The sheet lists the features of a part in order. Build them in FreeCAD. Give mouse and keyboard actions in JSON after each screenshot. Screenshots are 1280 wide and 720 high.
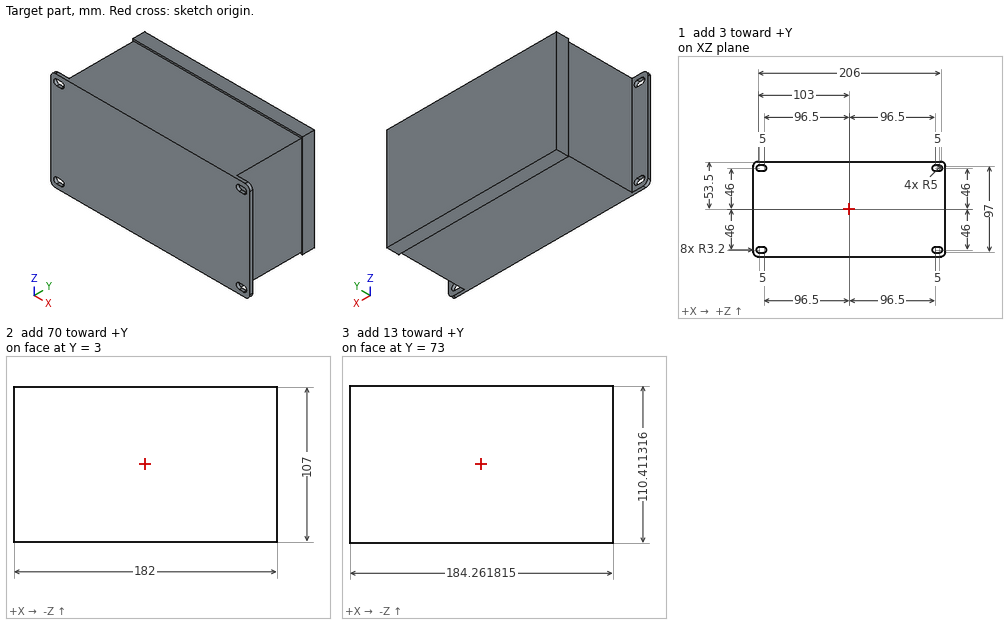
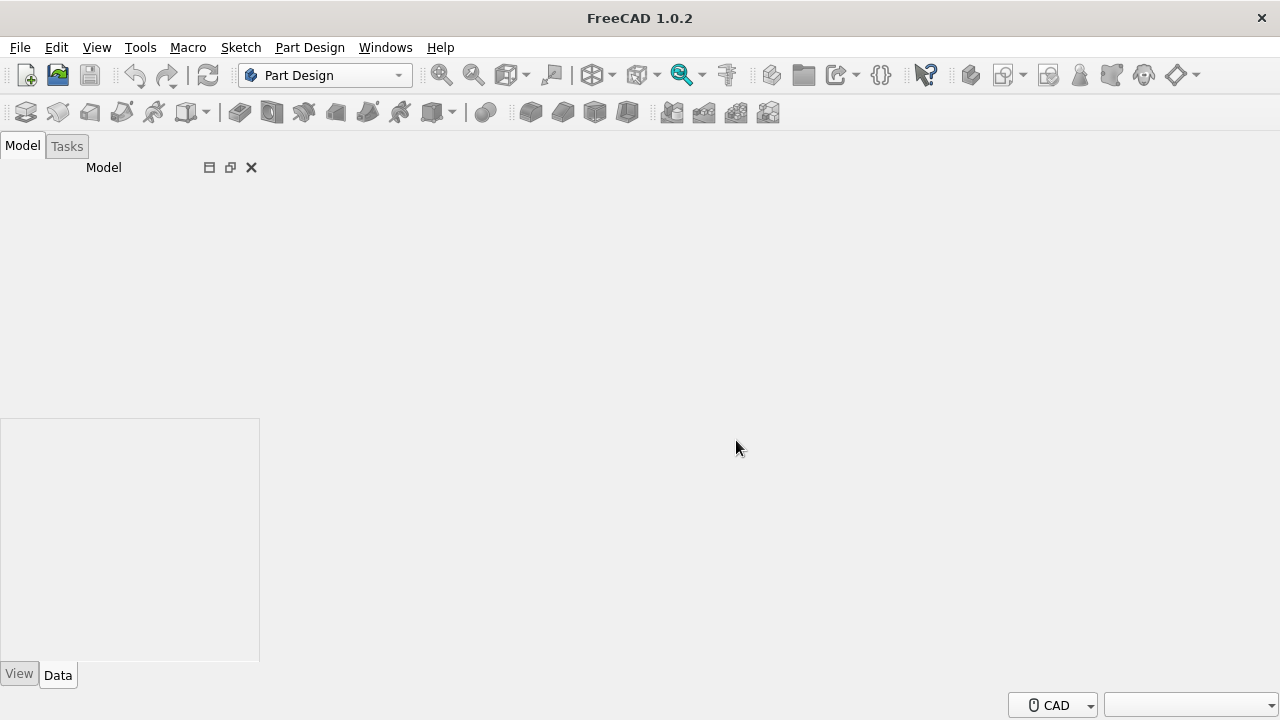
{"action": "left_click", "coordinate": [26, 76]}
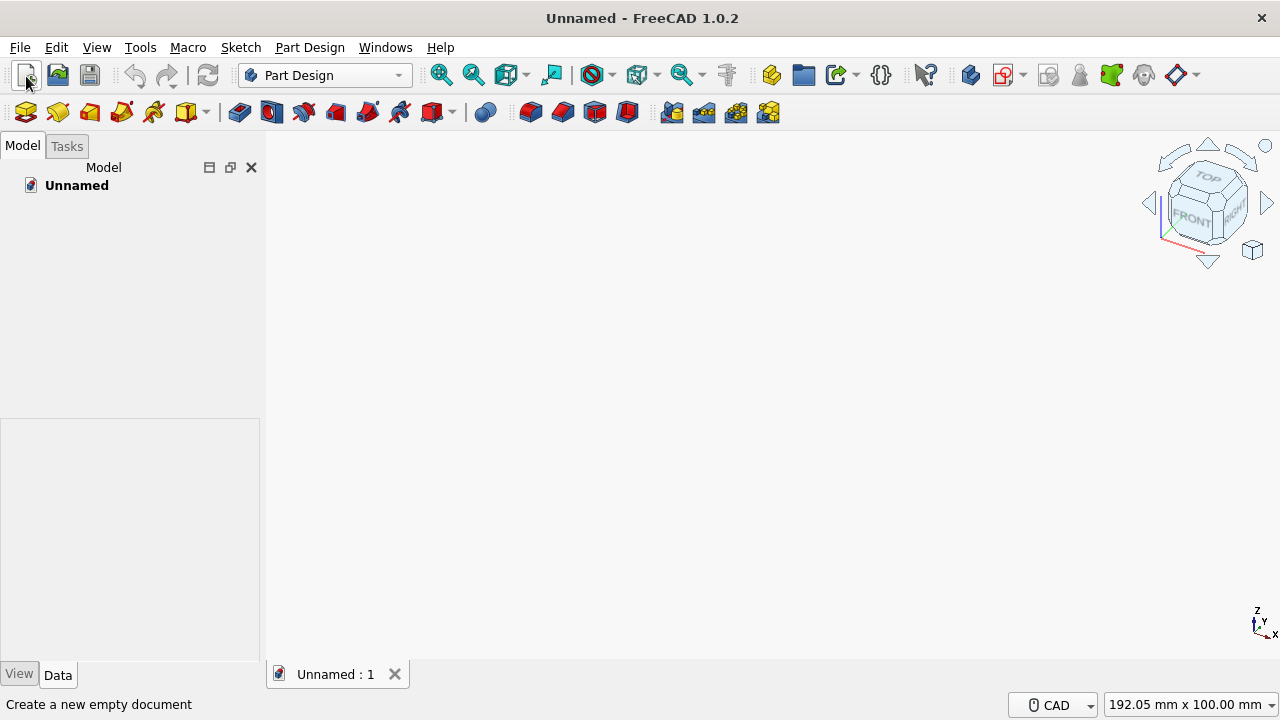
{"action": "left_click", "coordinate": [1004, 76]}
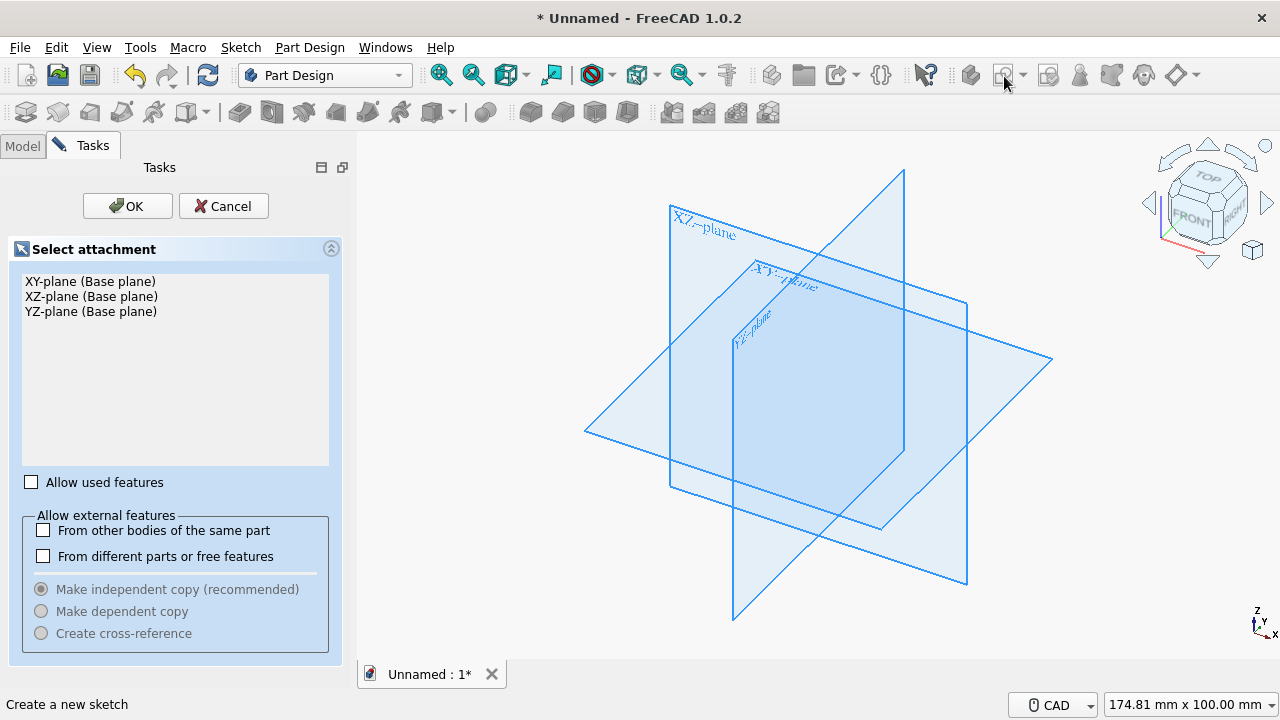
{"action": "left_click", "coordinate": [82, 296]}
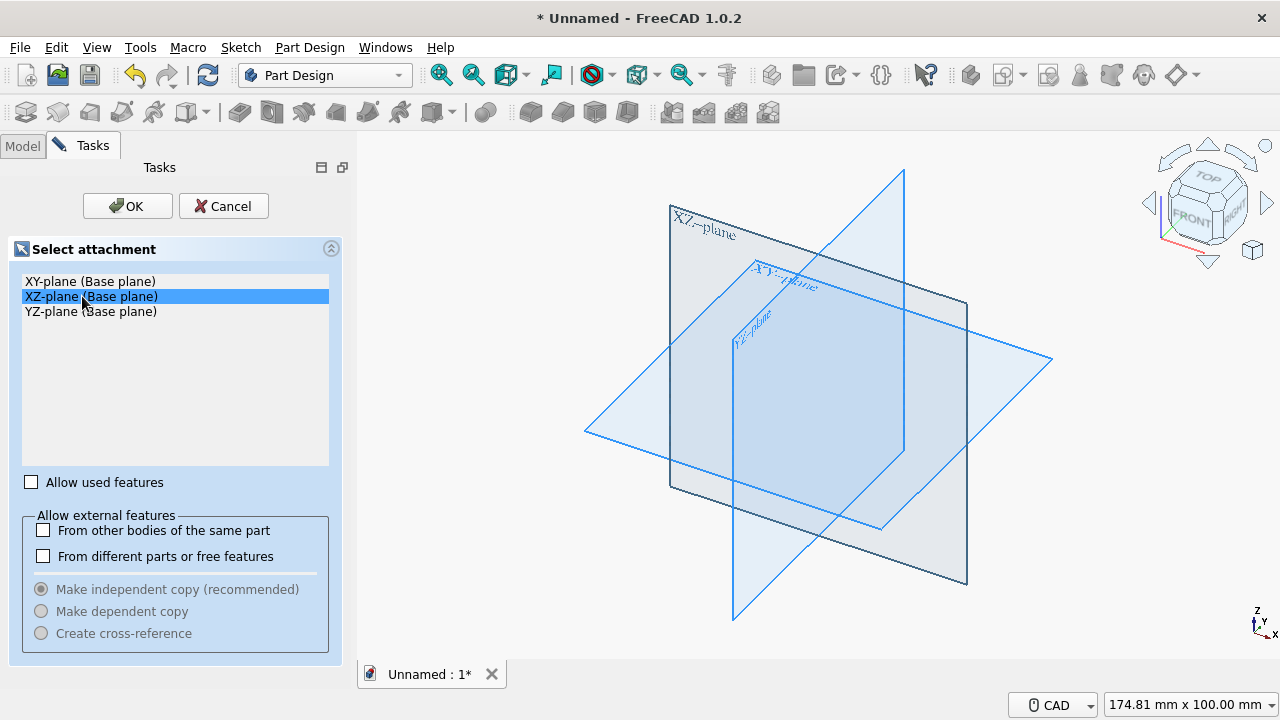
{"action": "left_click", "coordinate": [128, 206]}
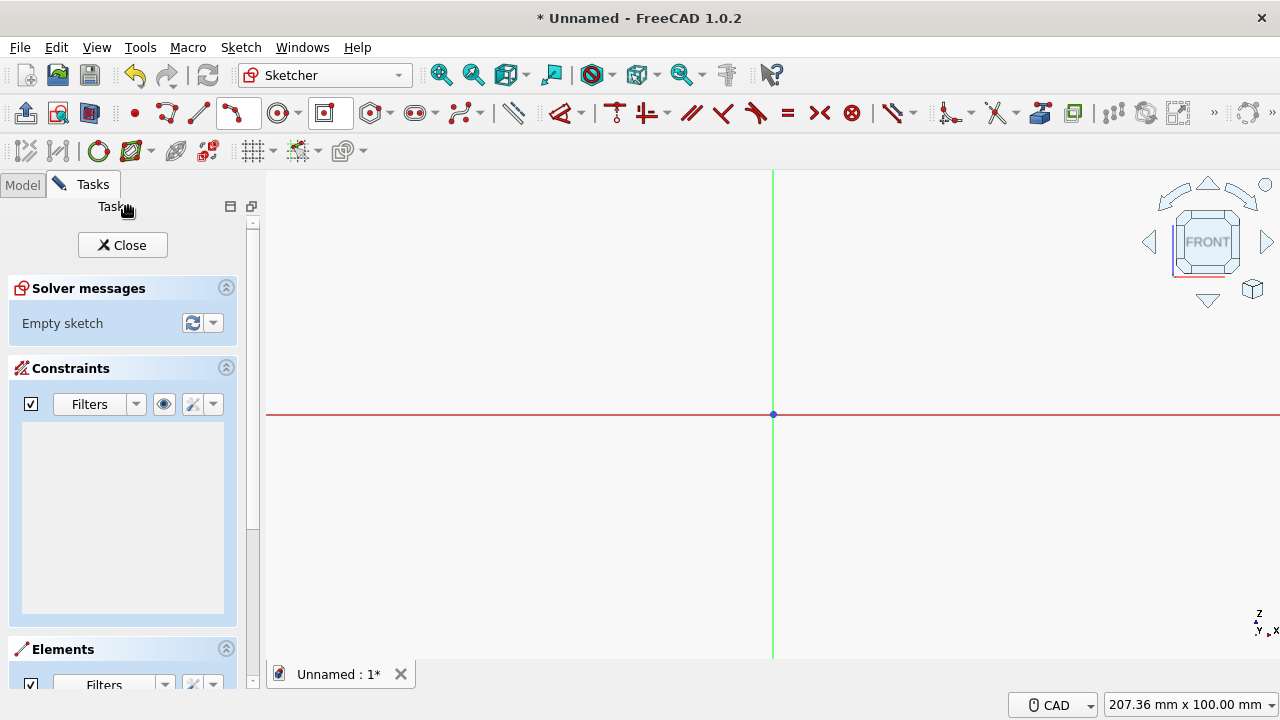
{"action": "scroll", "coordinate": [621, 414], "scroll_direction": "down", "scroll_amount": 3}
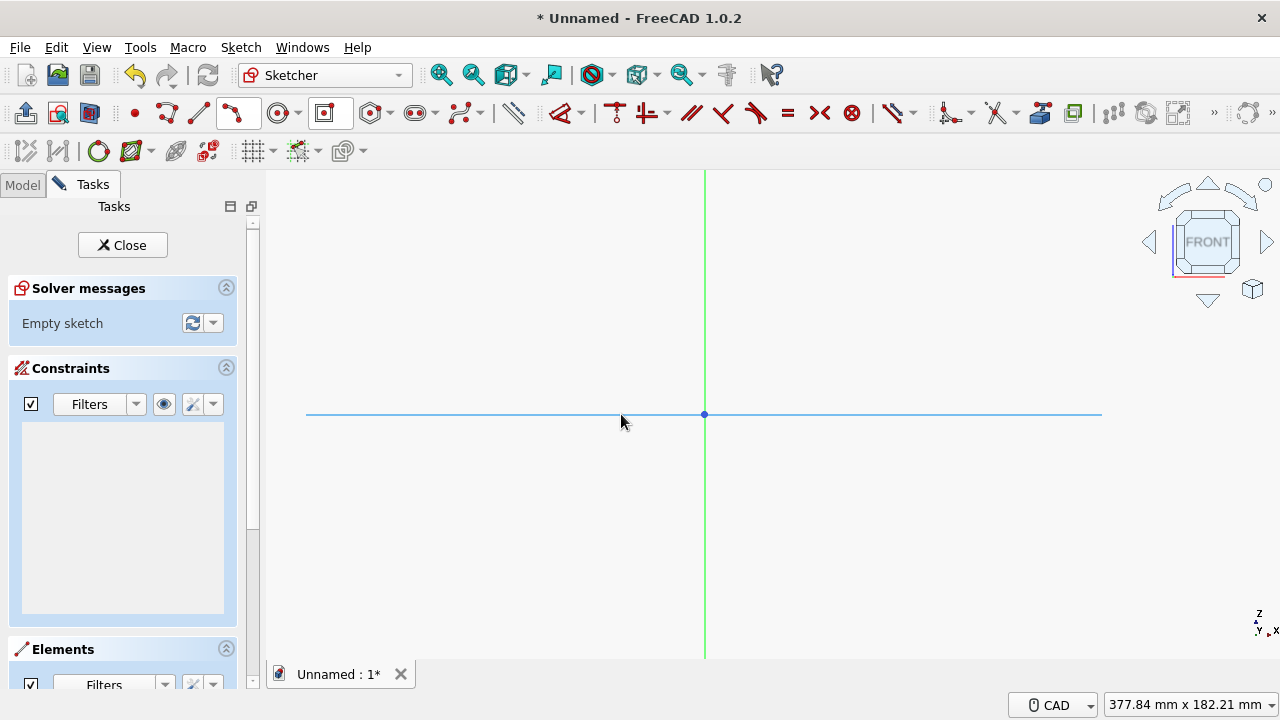
{"action": "left_click", "coordinate": [200, 114]}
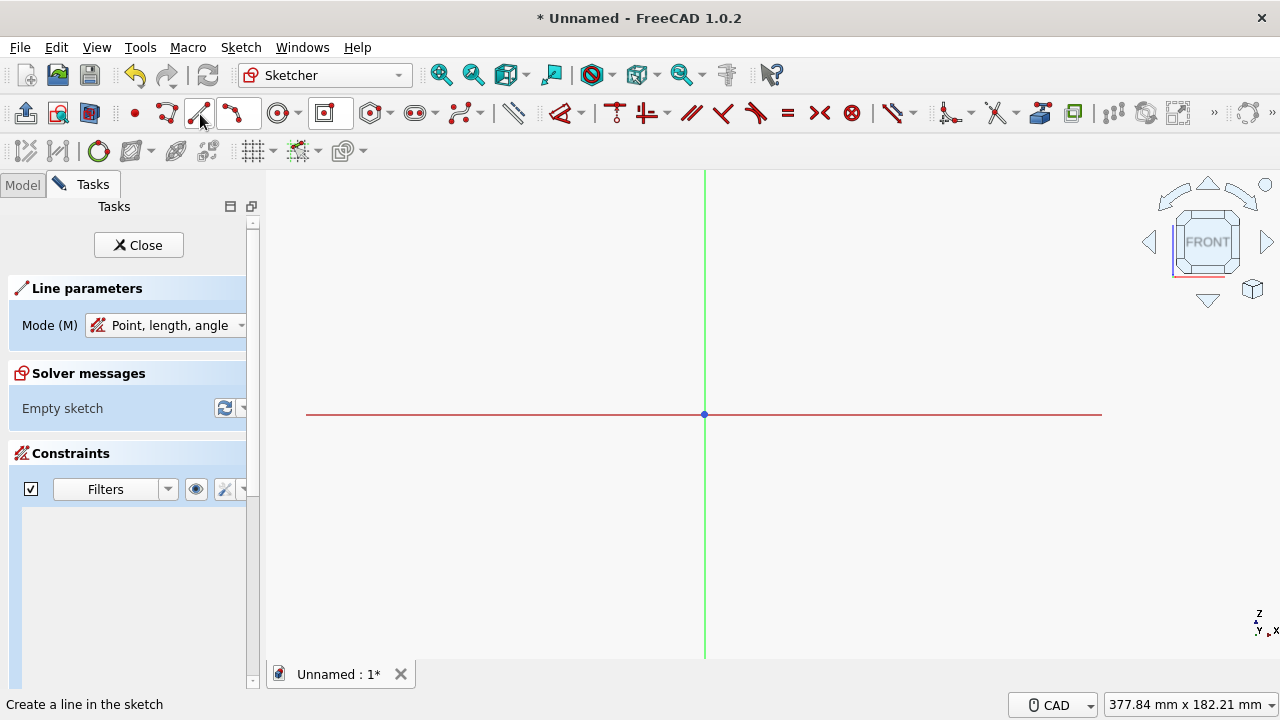
{"action": "left_click", "coordinate": [428, 271]}
{"action": "left_click", "coordinate": [981, 271]}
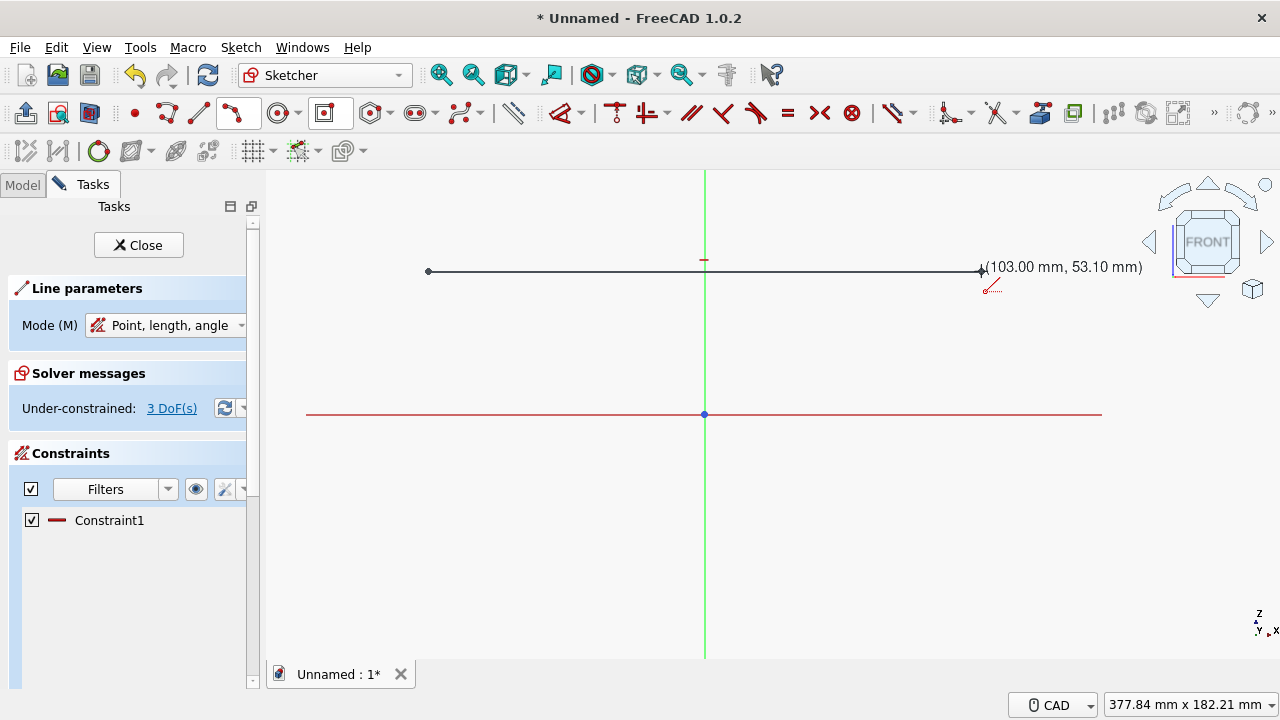
{"action": "left_click", "coordinate": [994, 284]}
{"action": "left_click", "coordinate": [994, 545]}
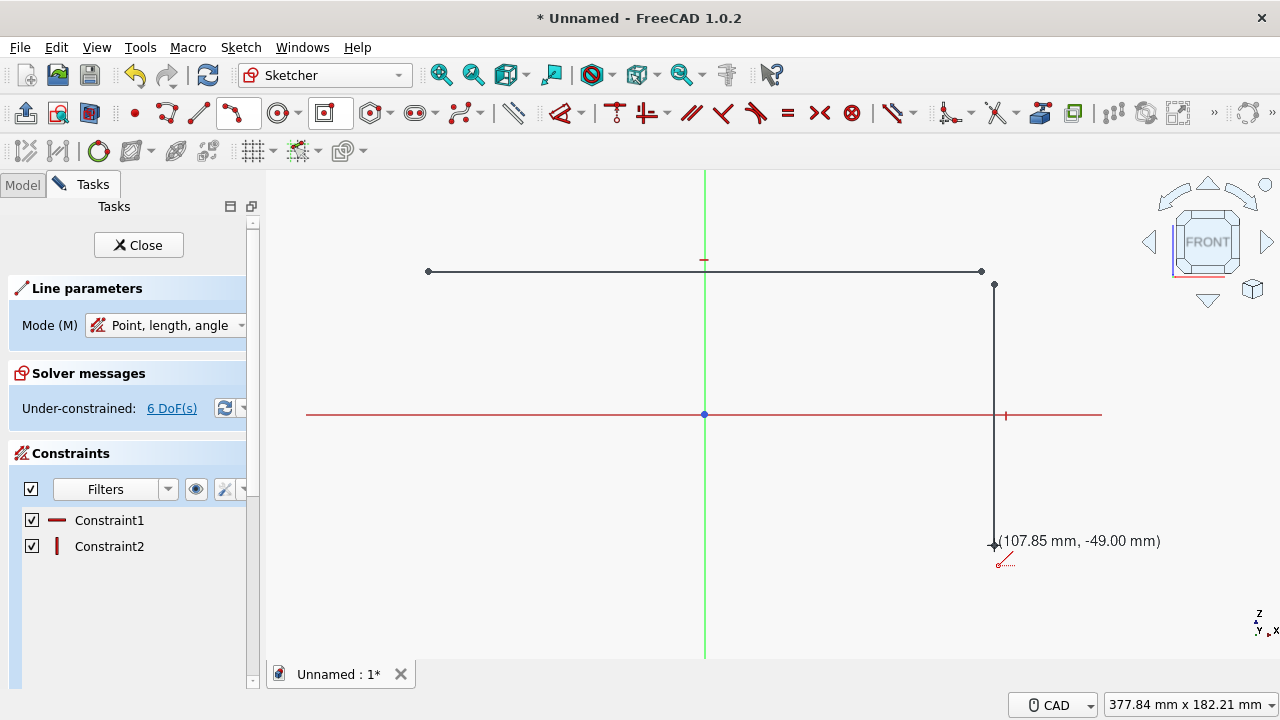
{"action": "left_click", "coordinate": [981, 558]}
{"action": "left_click", "coordinate": [428, 558]}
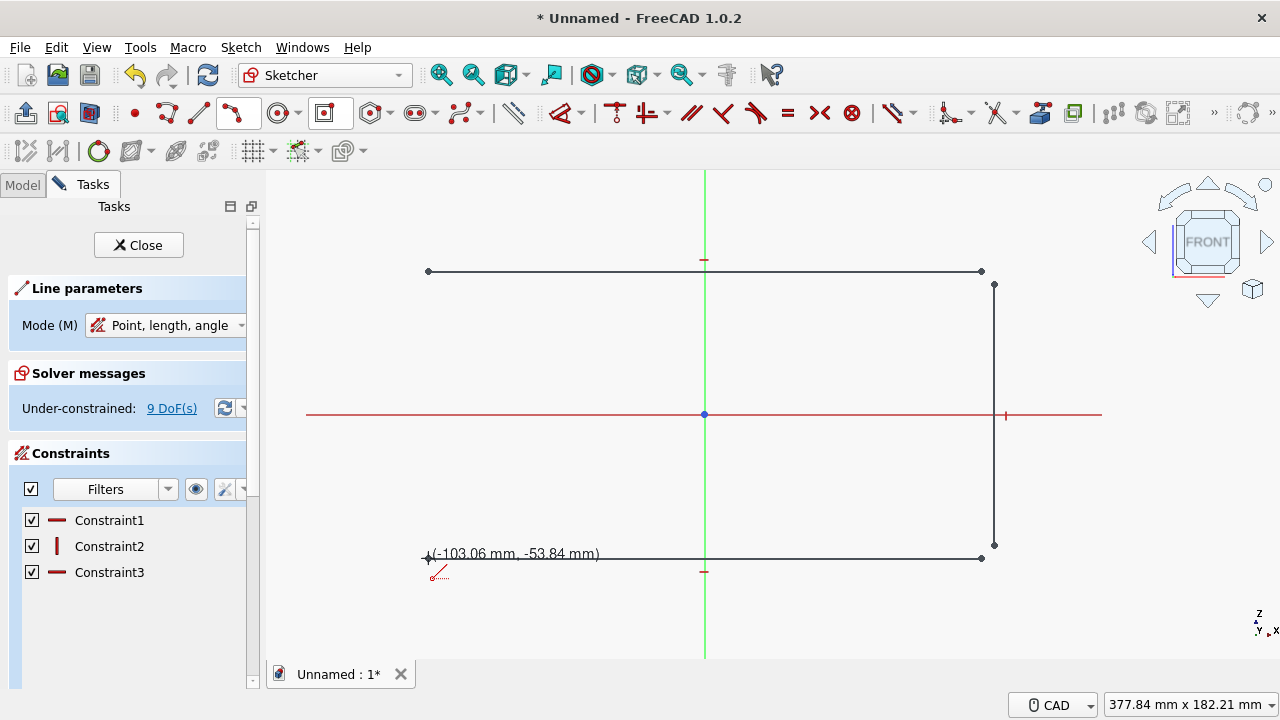
{"action": "left_click", "coordinate": [415, 545]}
{"action": "left_click", "coordinate": [415, 284]}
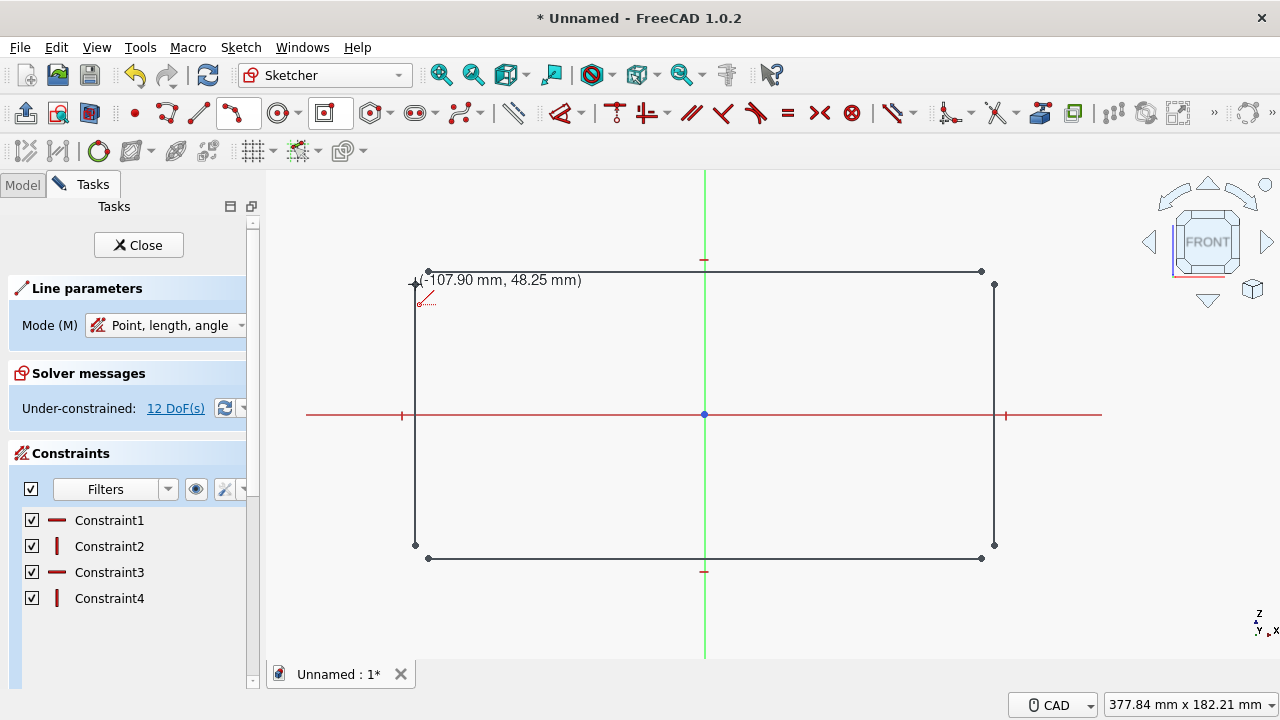
{"action": "left_click", "coordinate": [232, 114]}